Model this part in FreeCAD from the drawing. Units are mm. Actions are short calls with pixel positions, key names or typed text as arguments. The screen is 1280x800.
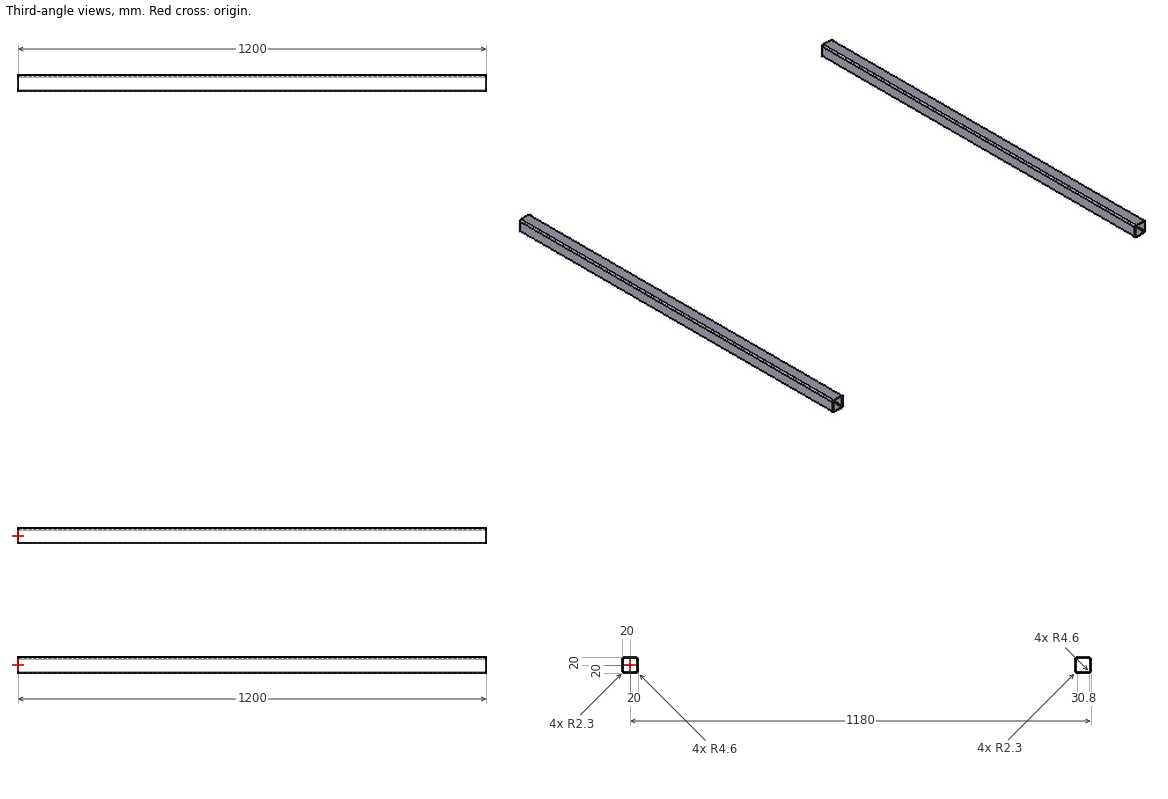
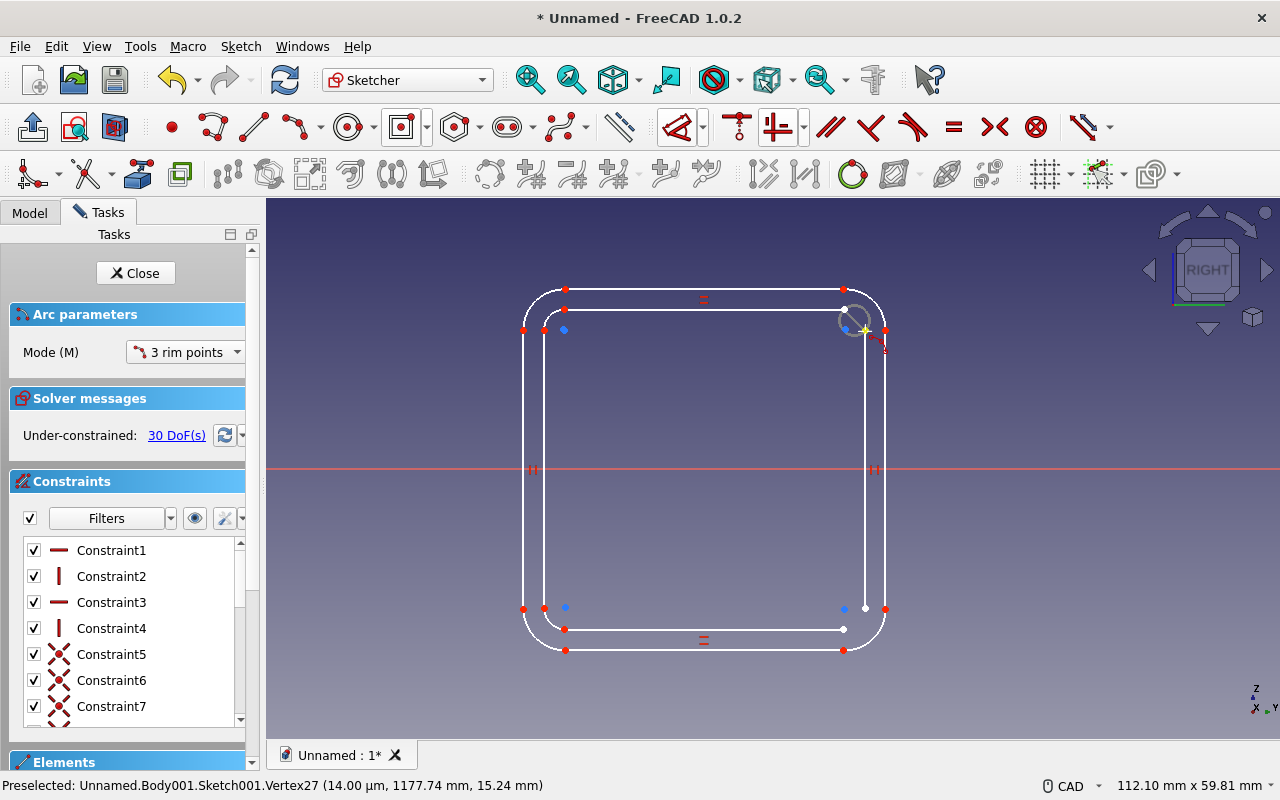
scroll(859, 315, up, 5)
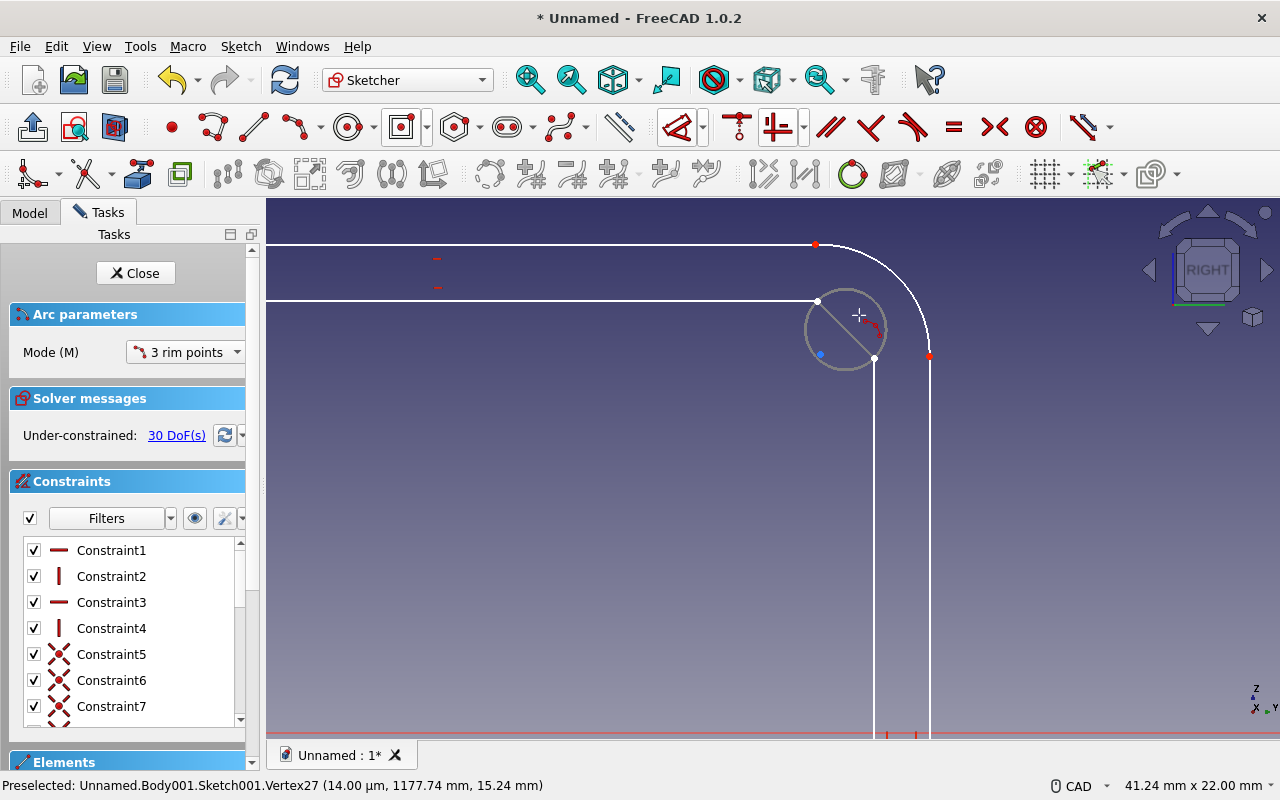
click(857, 314)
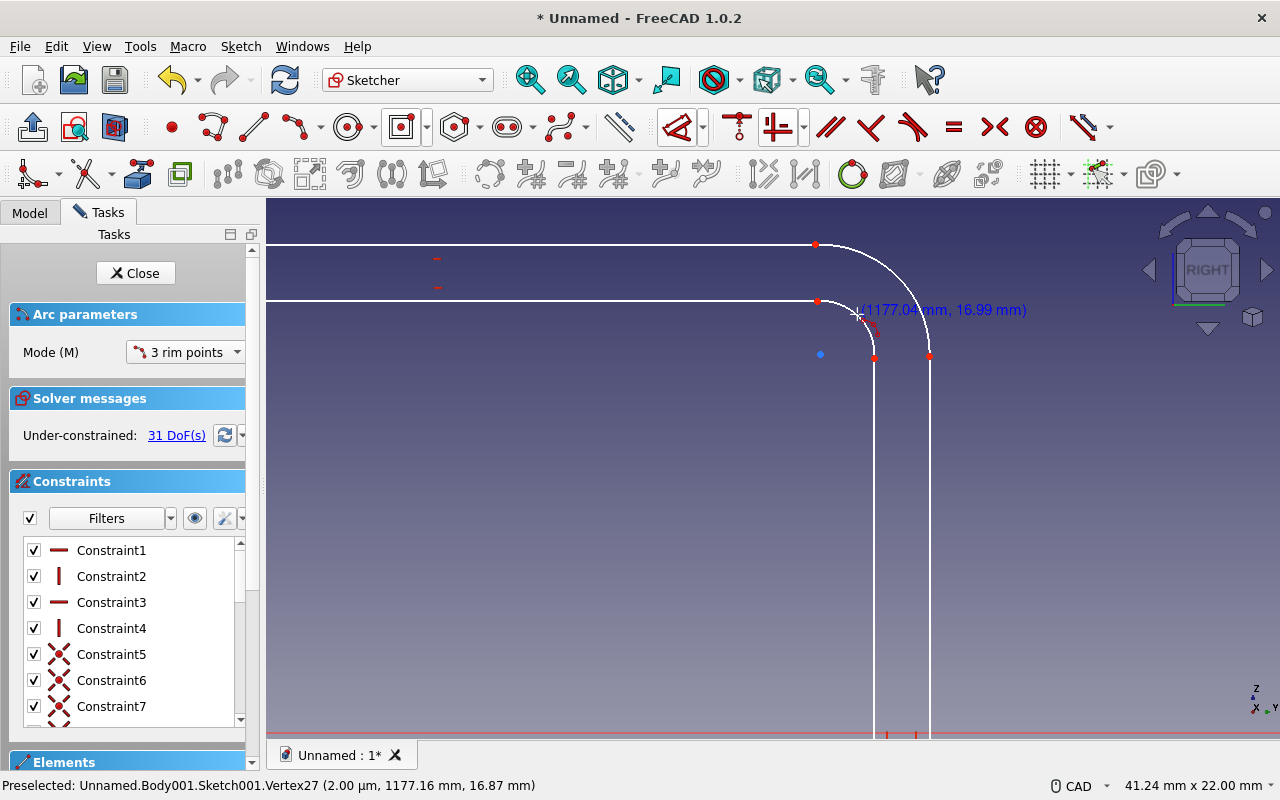
scroll(860, 315, down, 5)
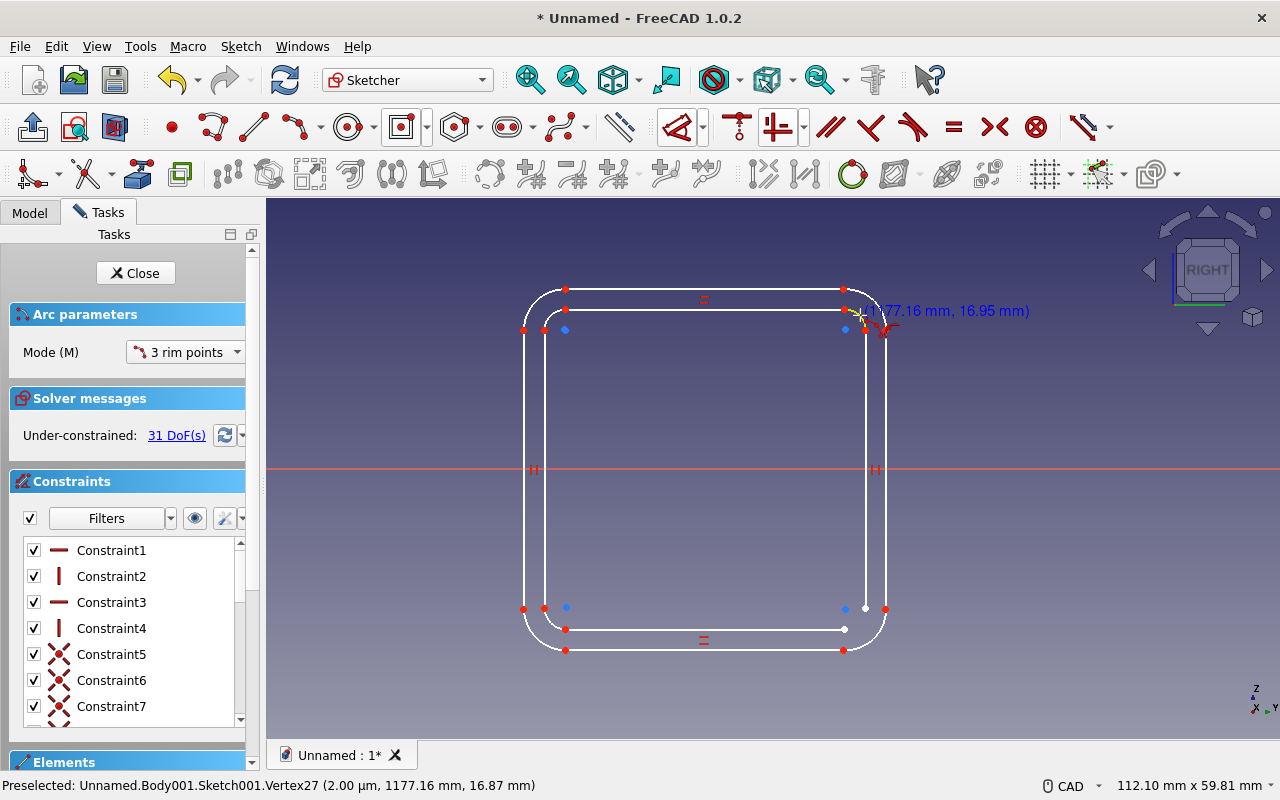
click(866, 609)
click(844, 630)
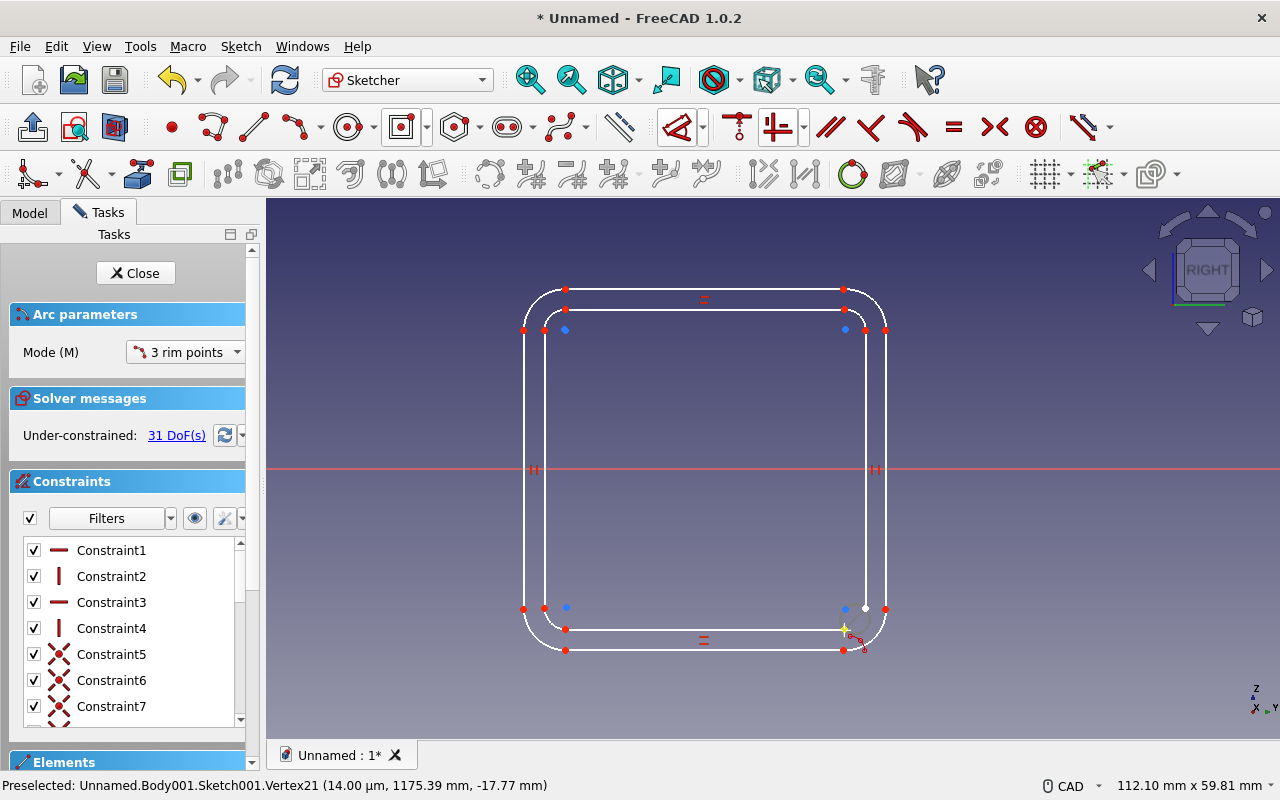
scroll(859, 623, up, 5)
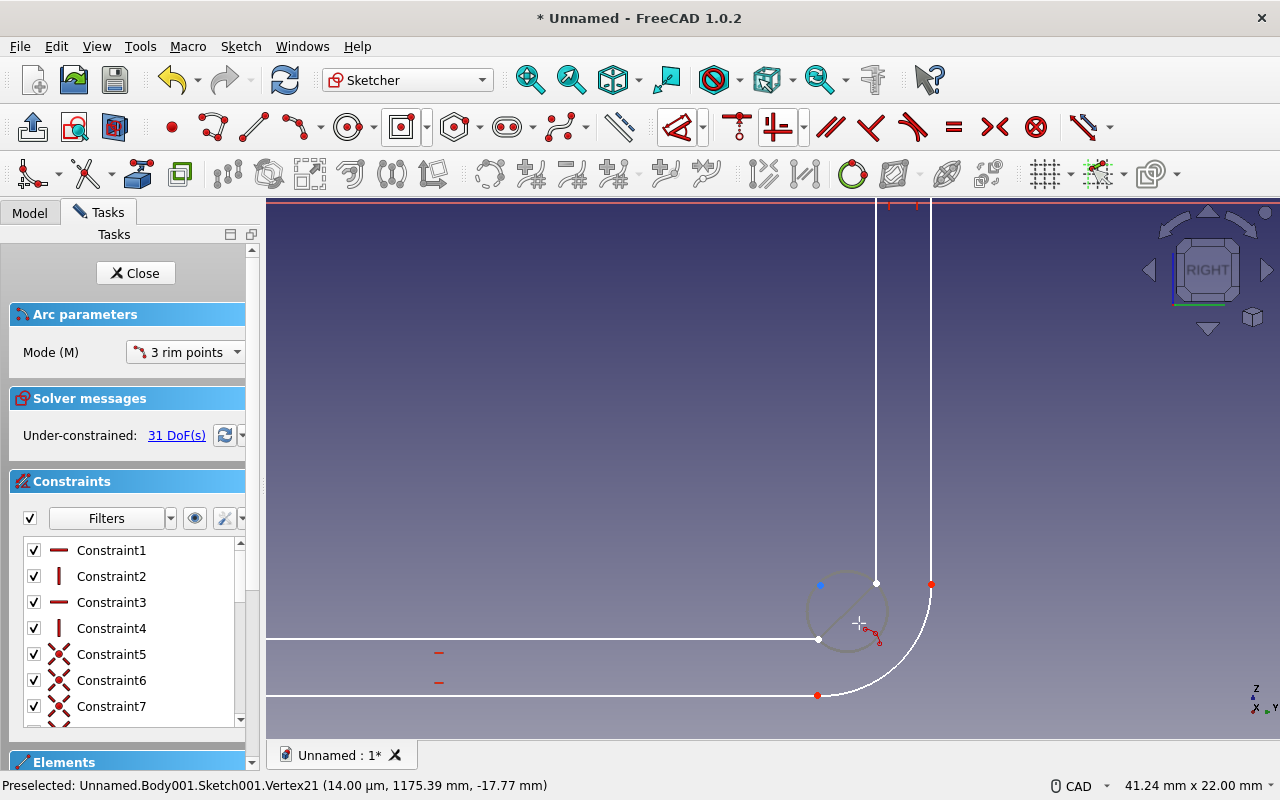
click(858, 621)
key(Escape)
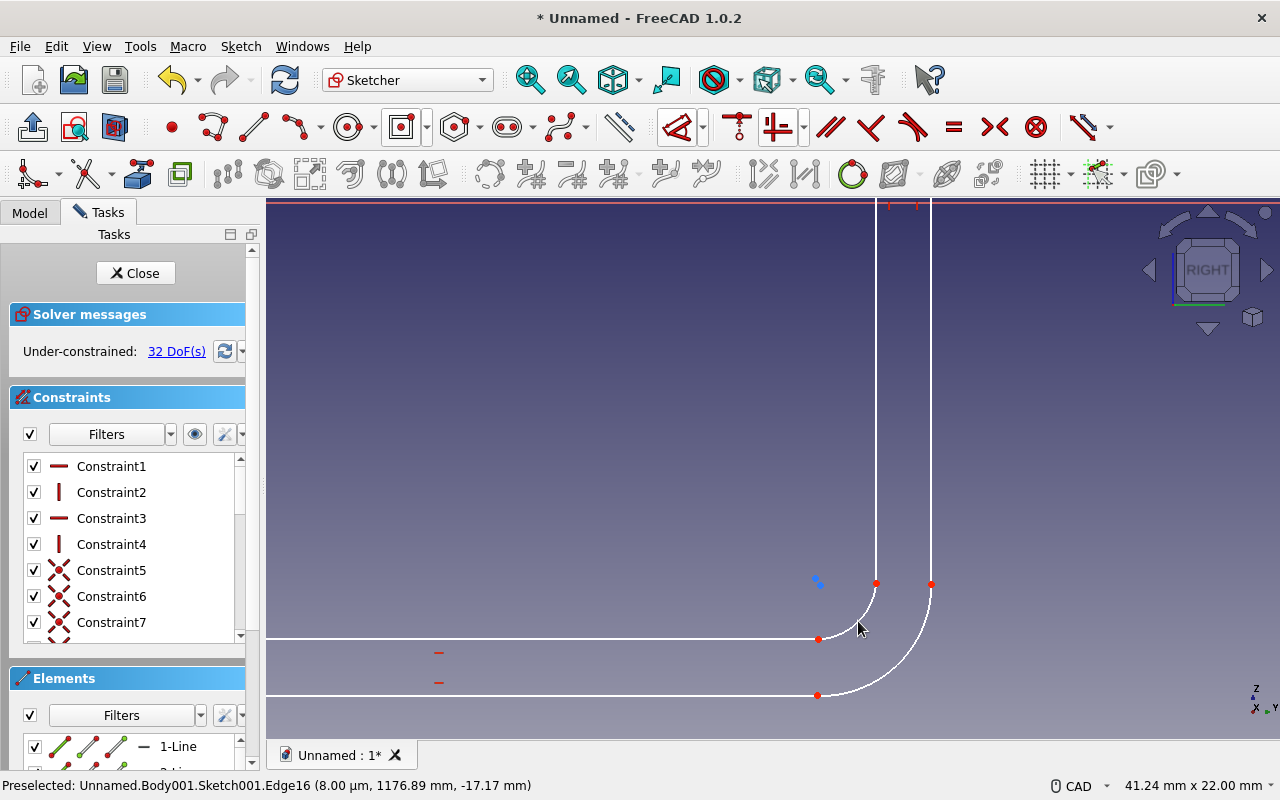
click(590, 696)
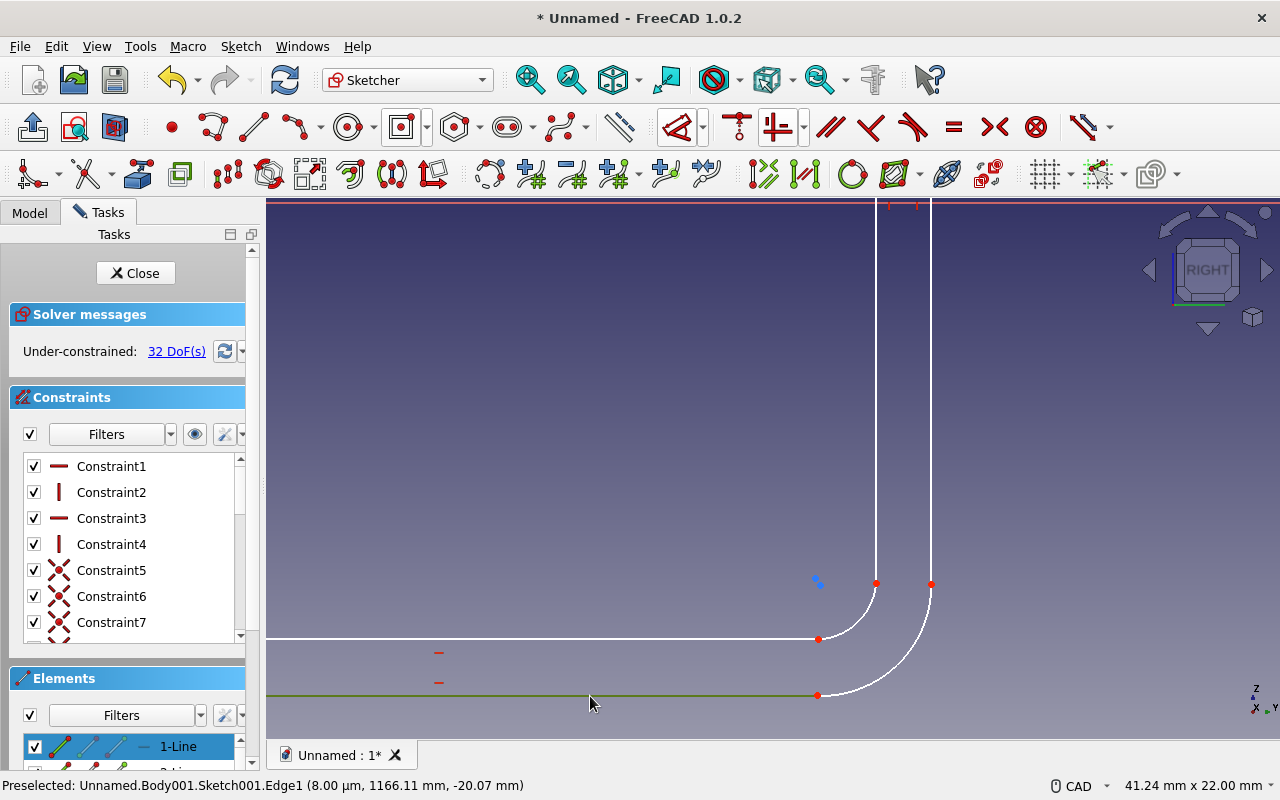
click(869, 685)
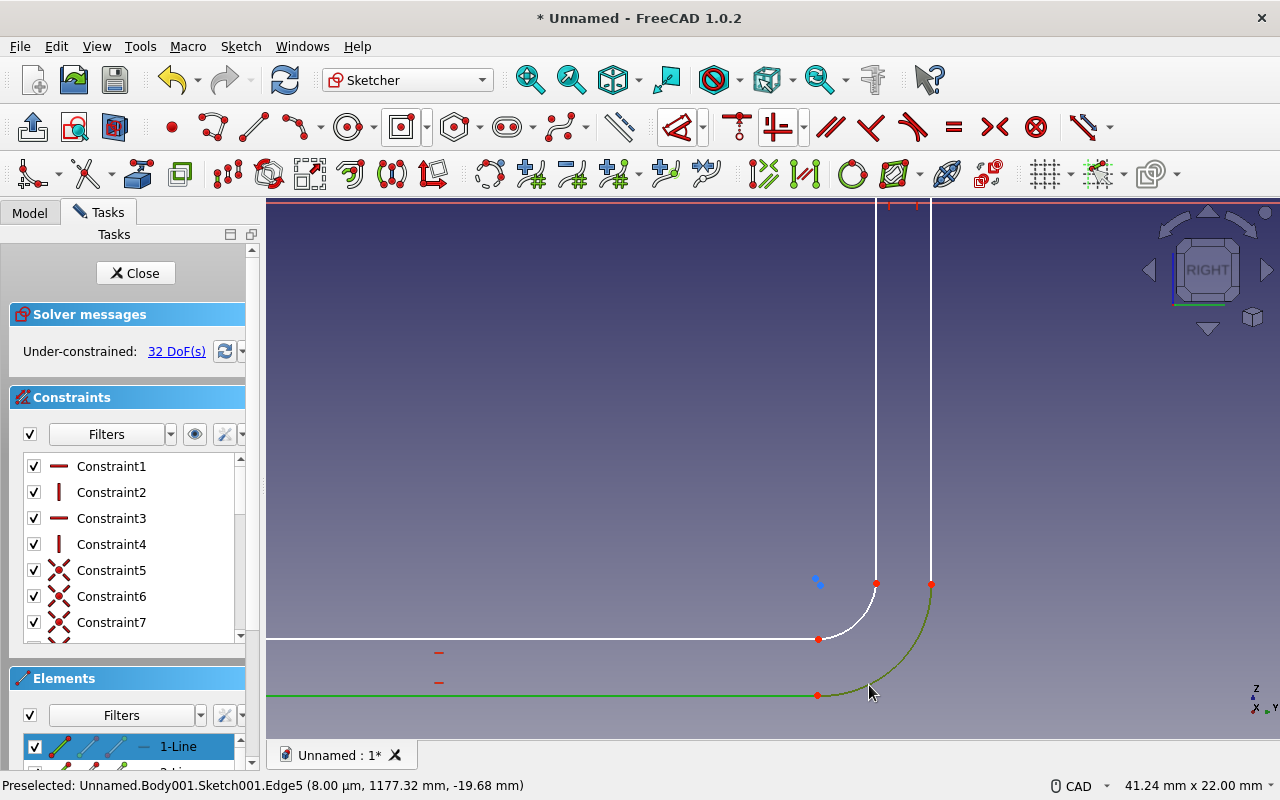
key(t)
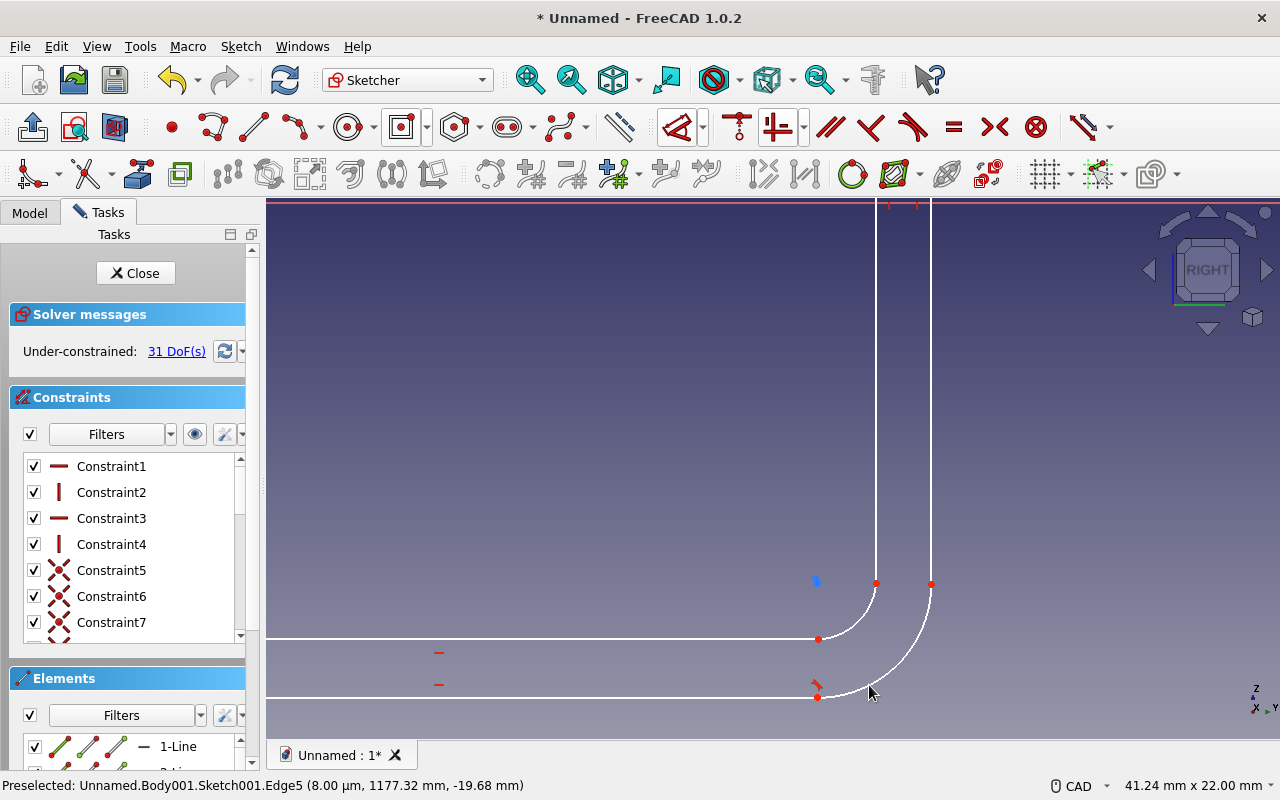
click(590, 698)